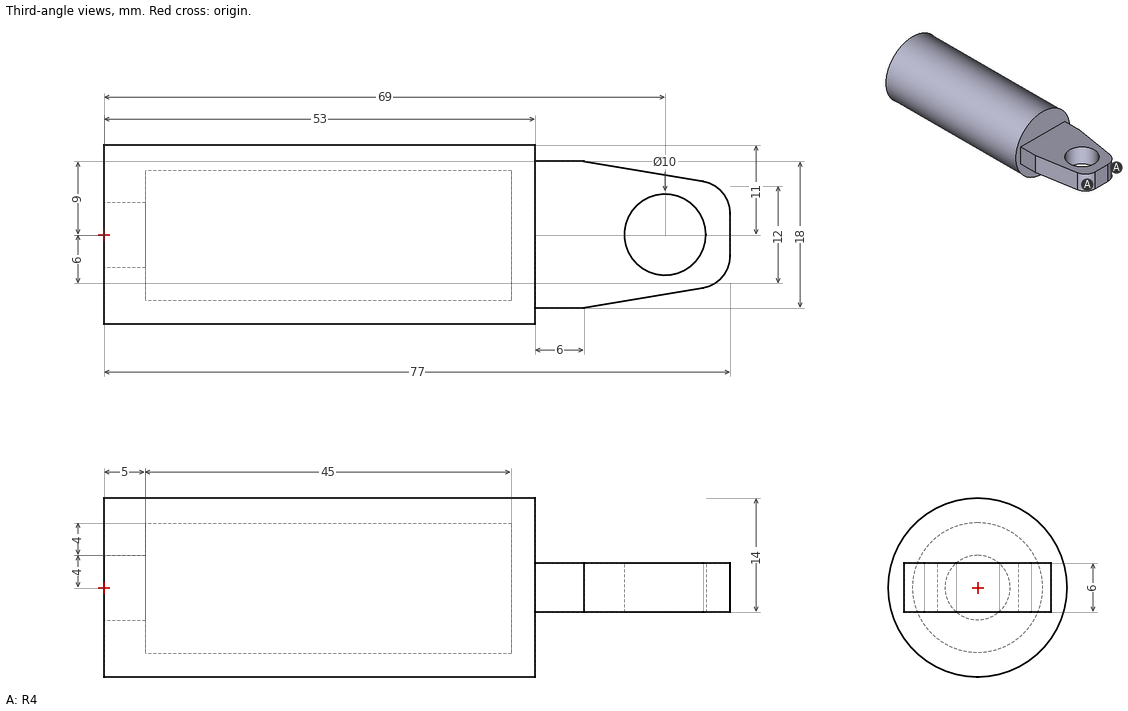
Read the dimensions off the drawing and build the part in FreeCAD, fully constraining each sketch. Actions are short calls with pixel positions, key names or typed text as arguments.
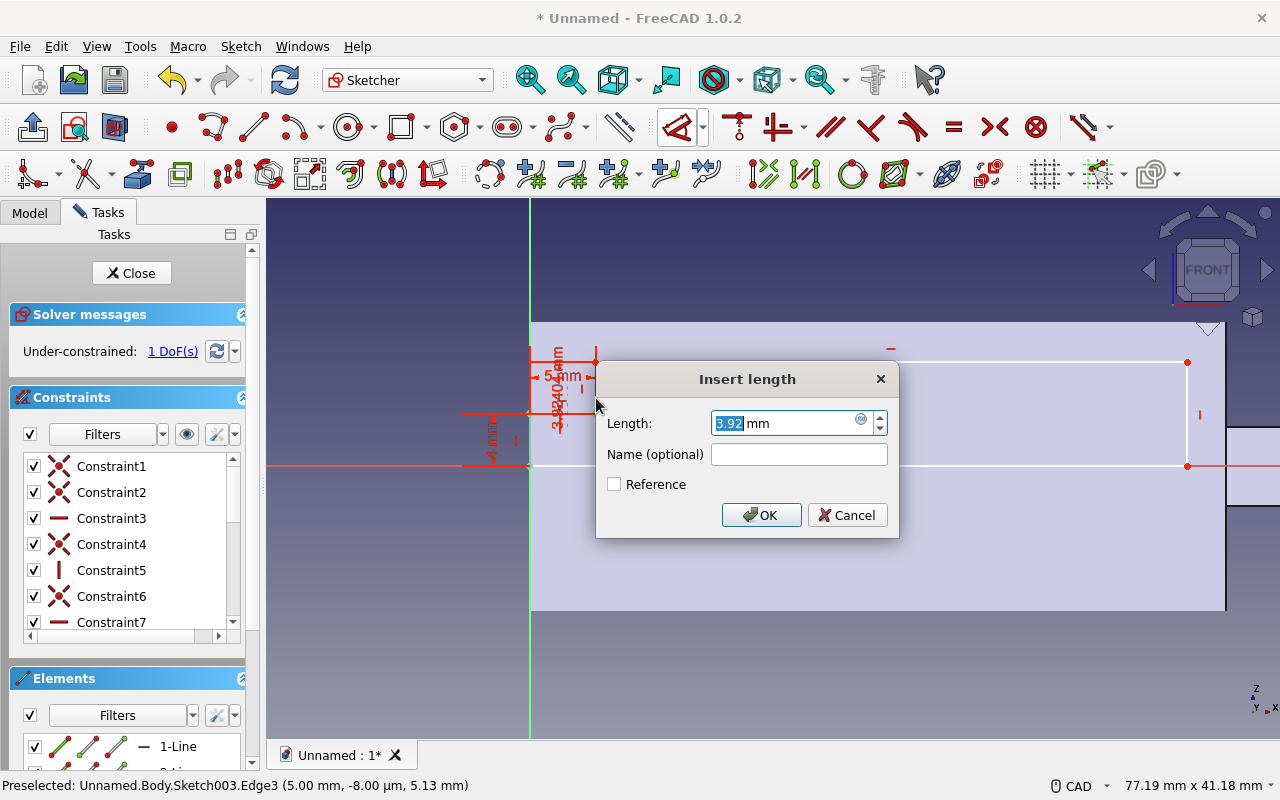
text(4)
key(Return)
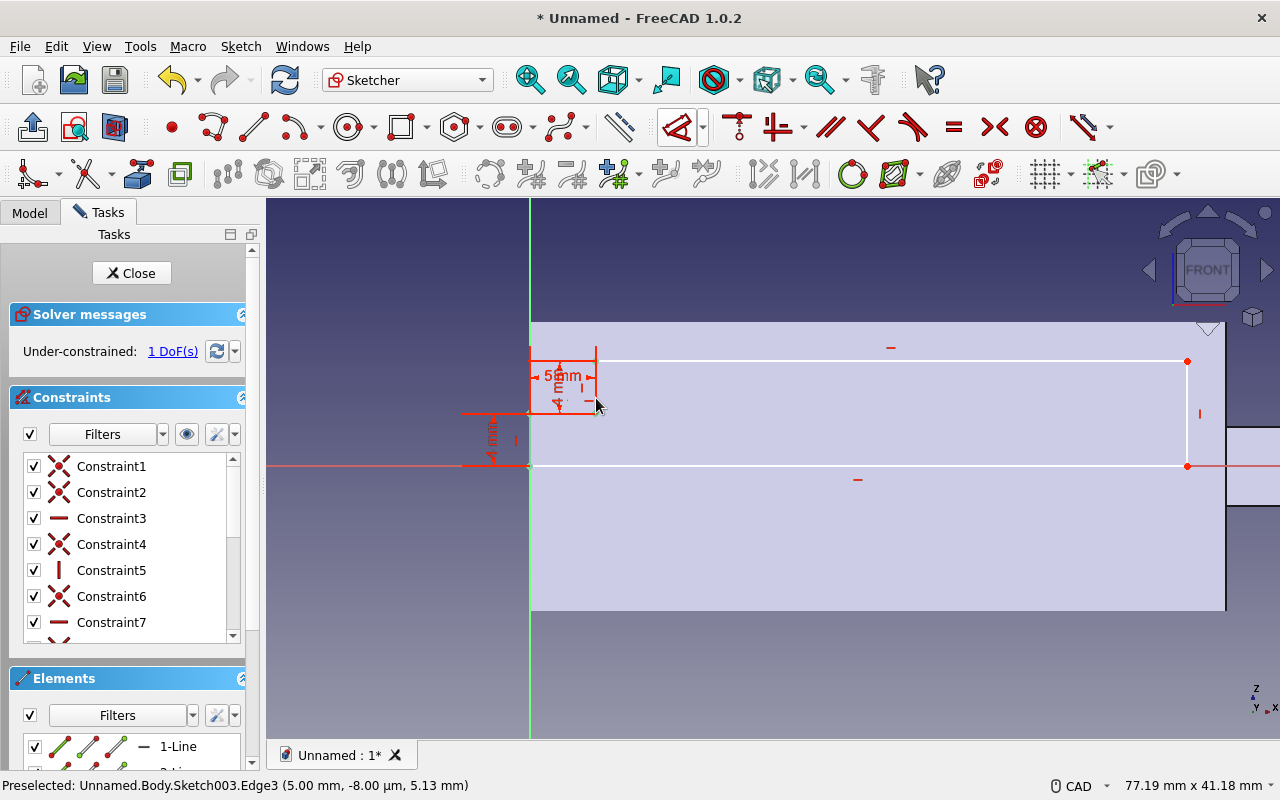
click(773, 361)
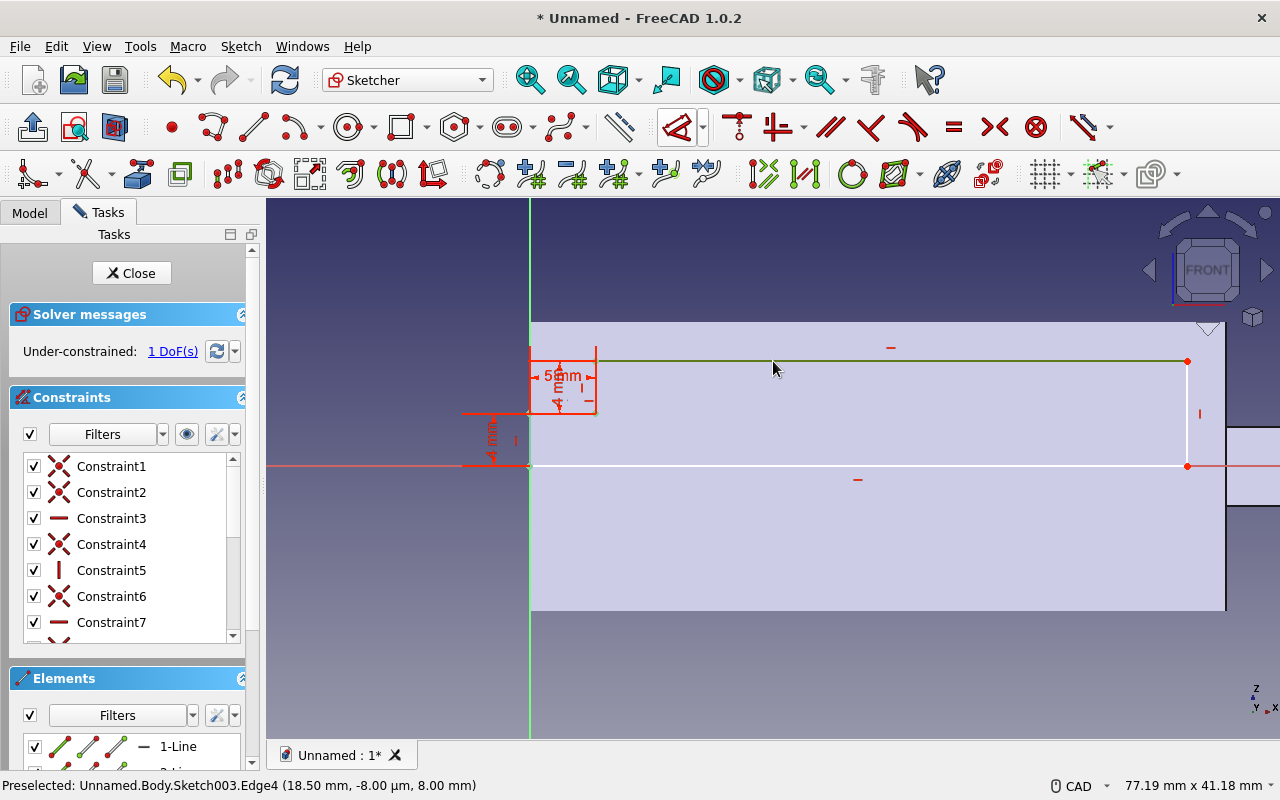
key(l)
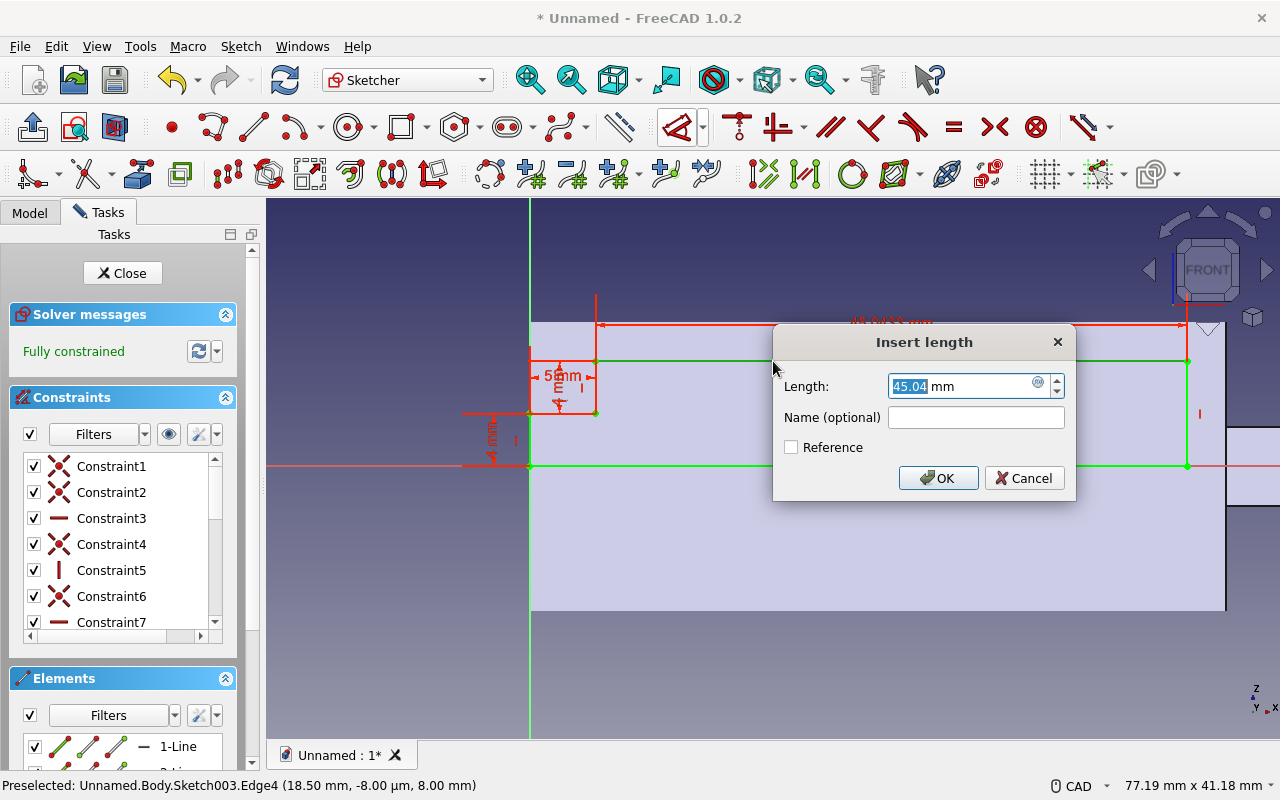
text(45)
key(Return)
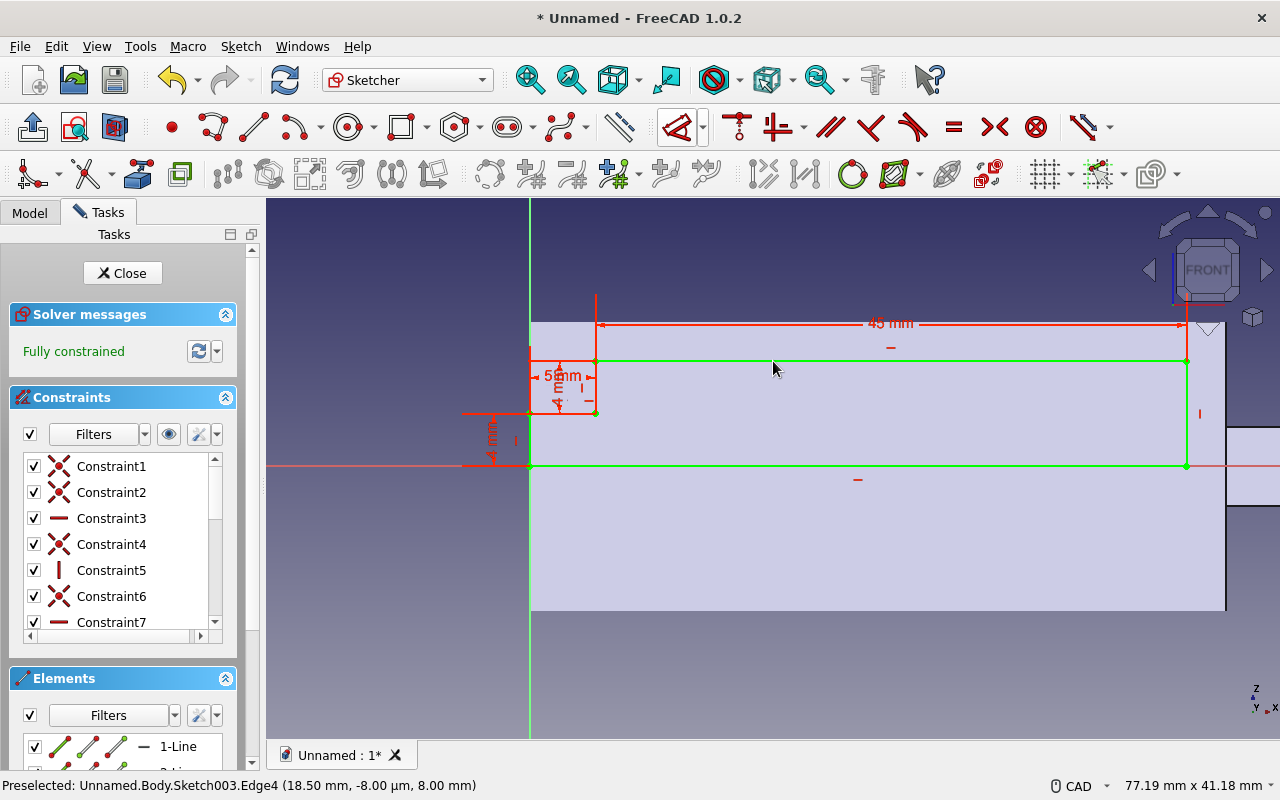
click(123, 273)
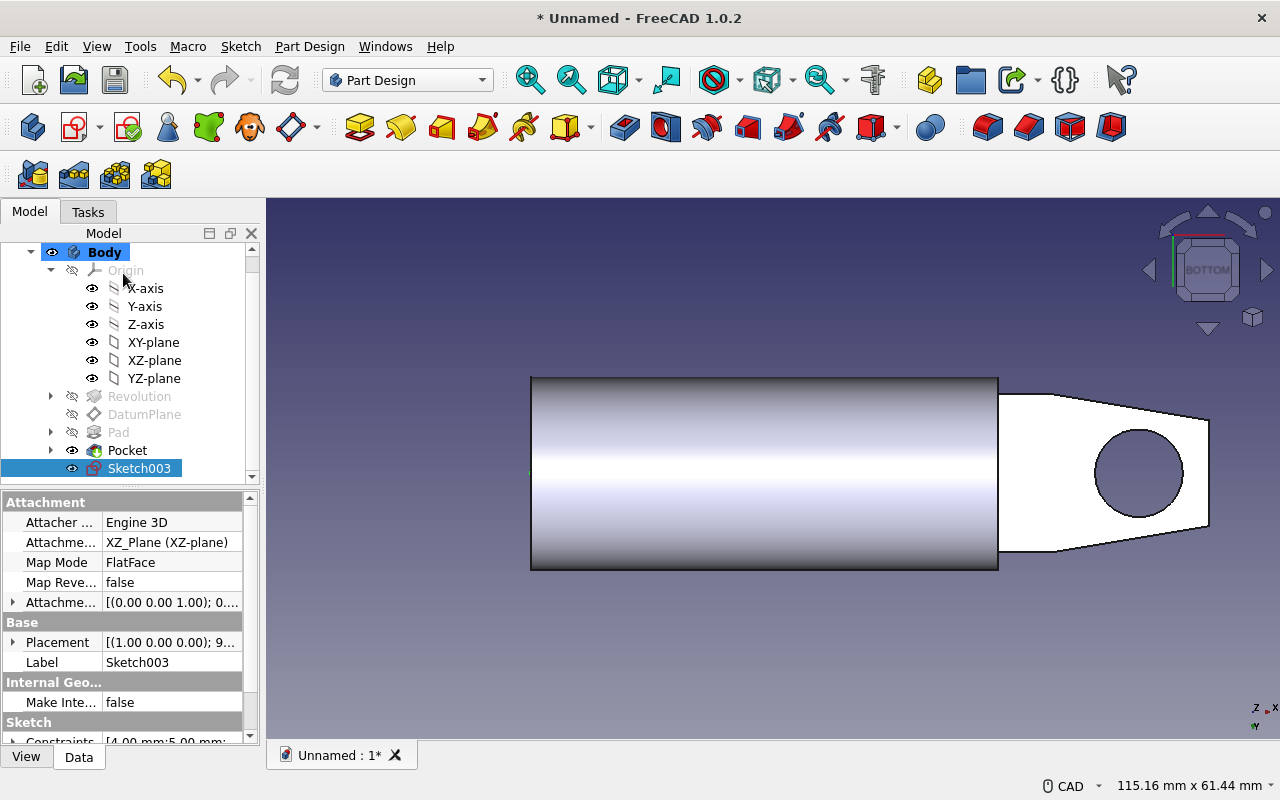
click(707, 128)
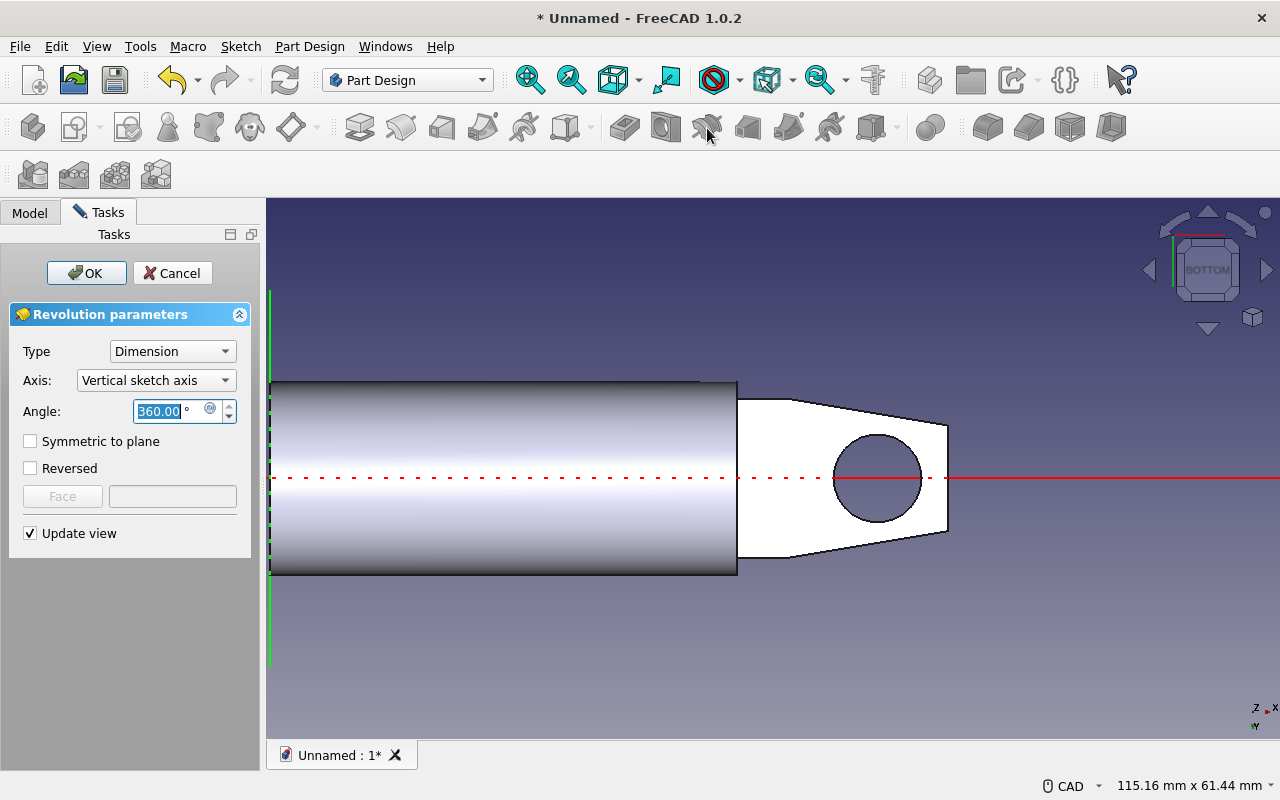
click(157, 380)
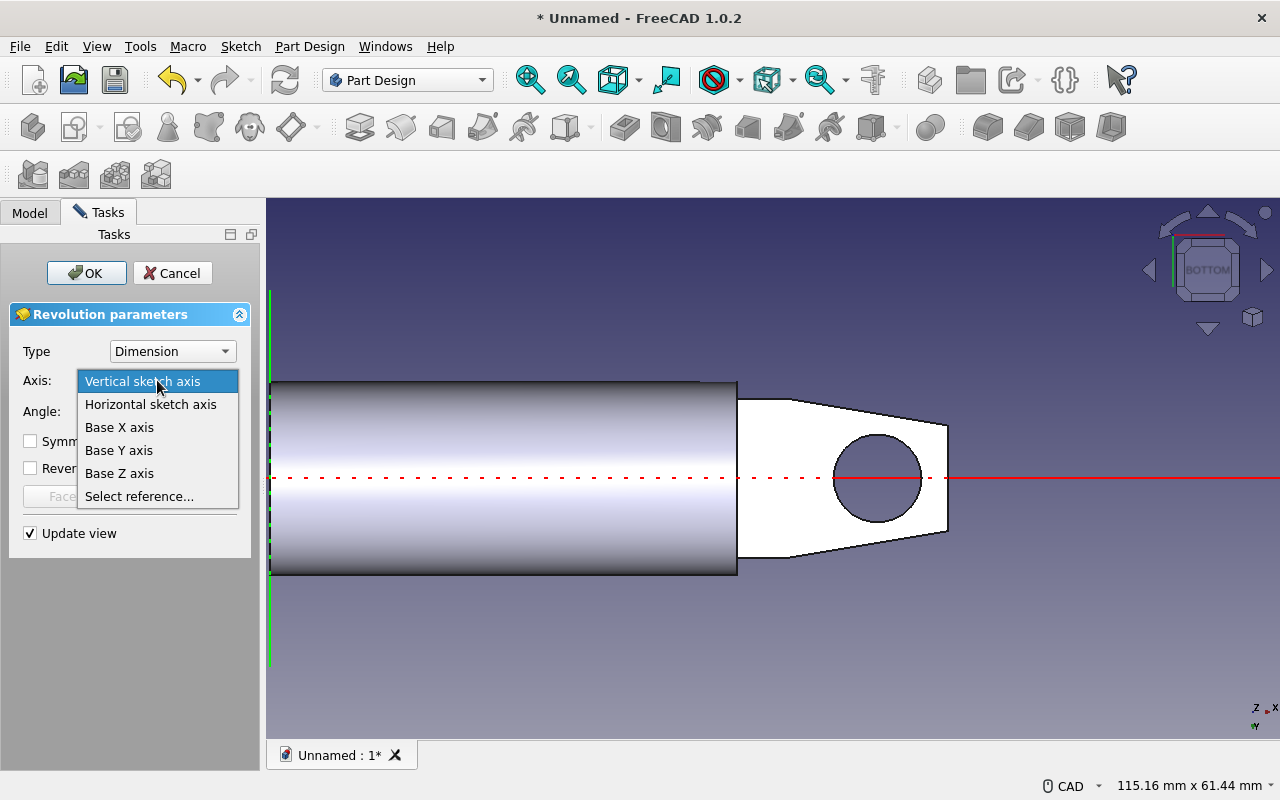
click(156, 404)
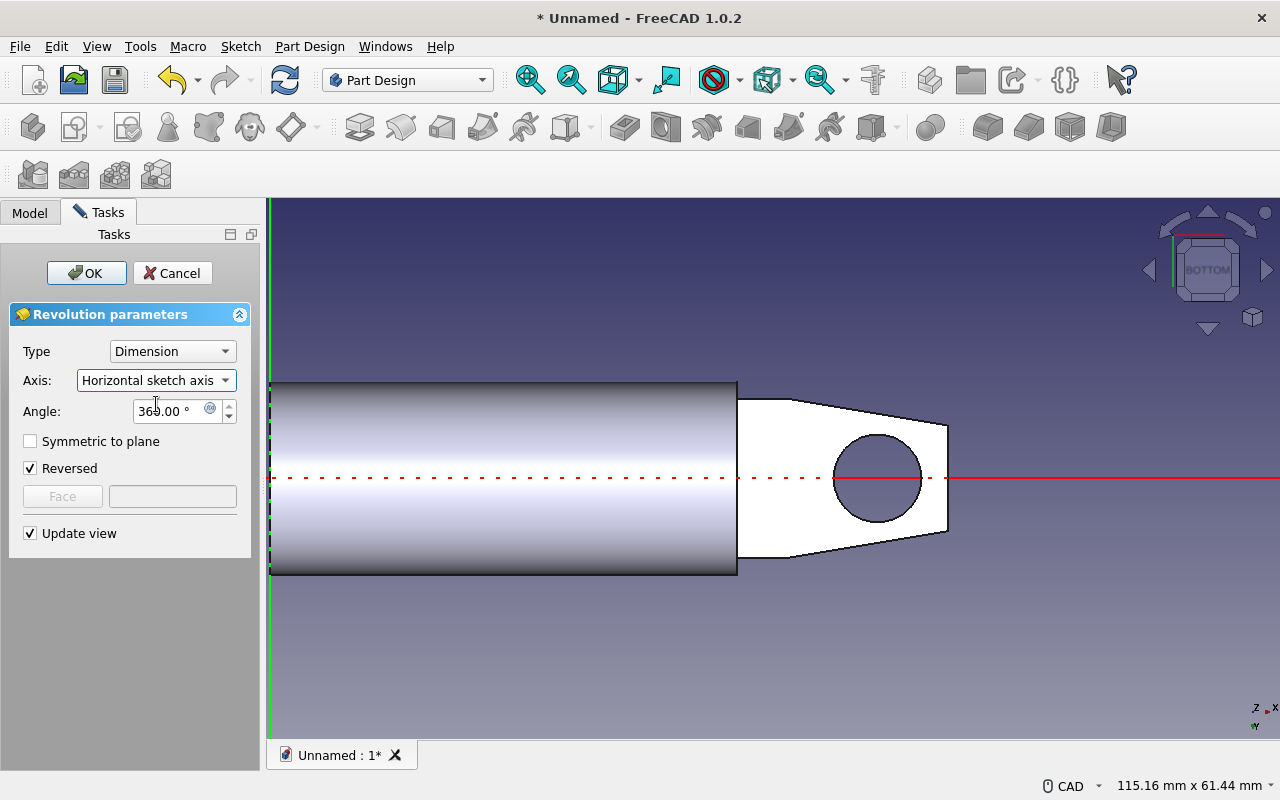
click(87, 273)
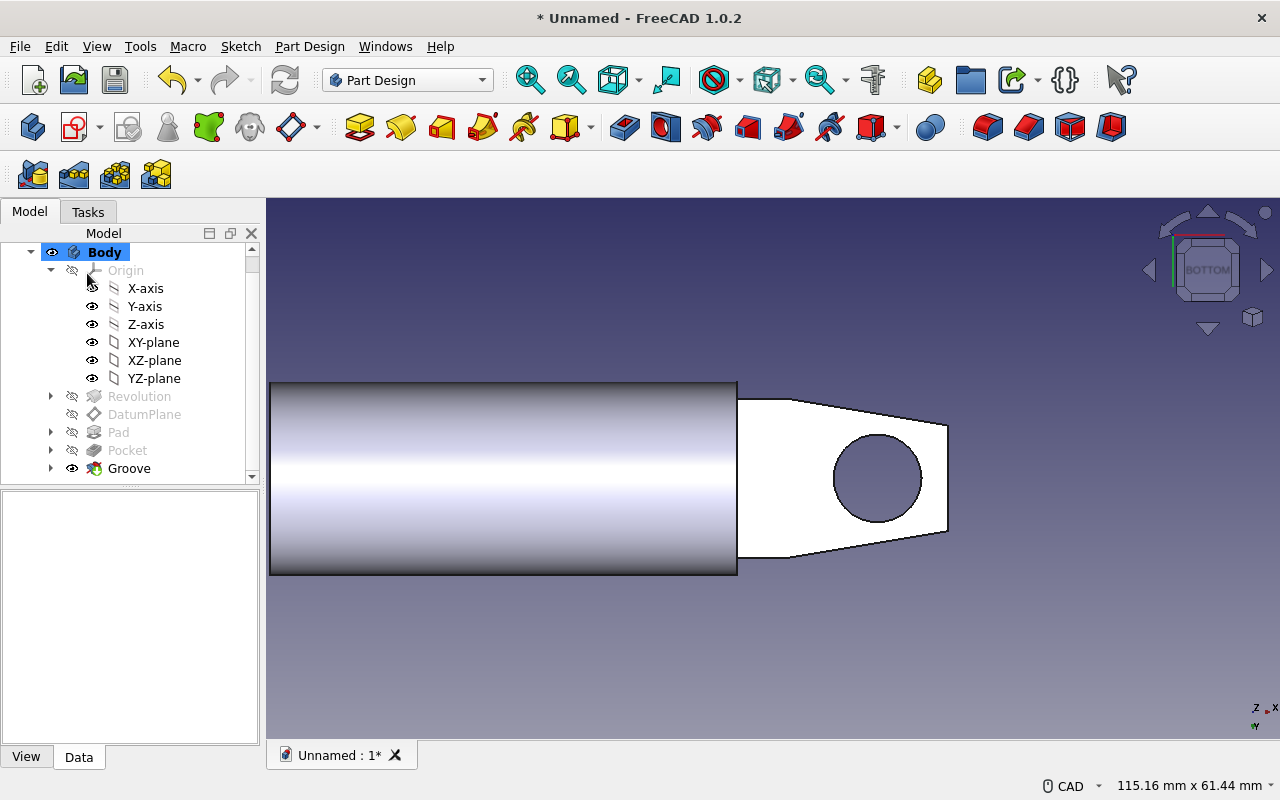
key(0)